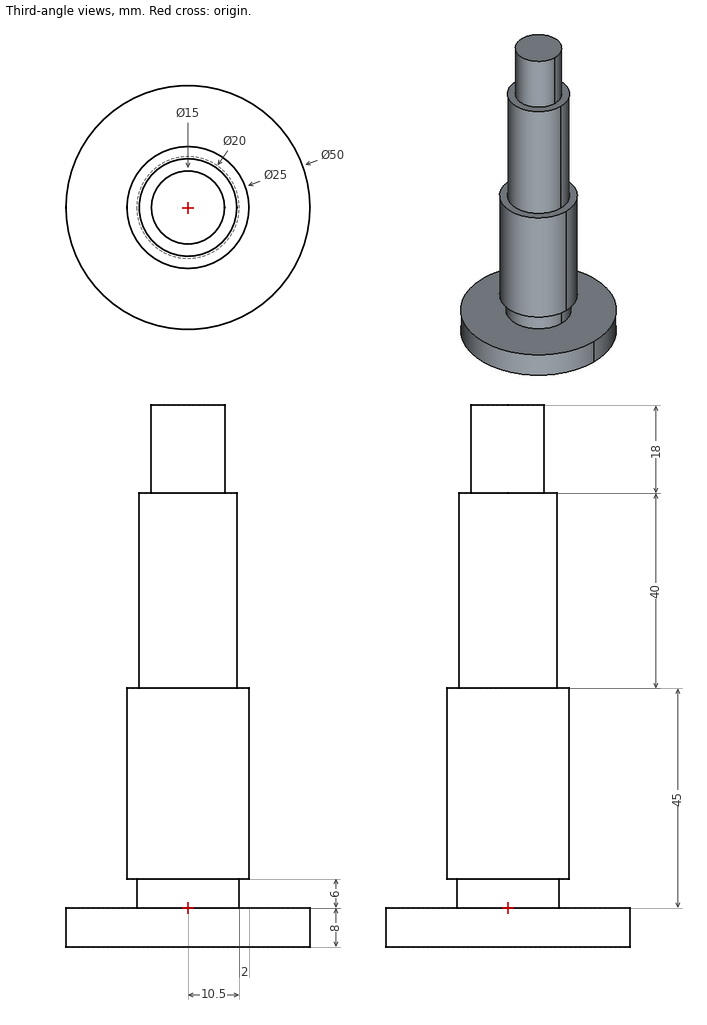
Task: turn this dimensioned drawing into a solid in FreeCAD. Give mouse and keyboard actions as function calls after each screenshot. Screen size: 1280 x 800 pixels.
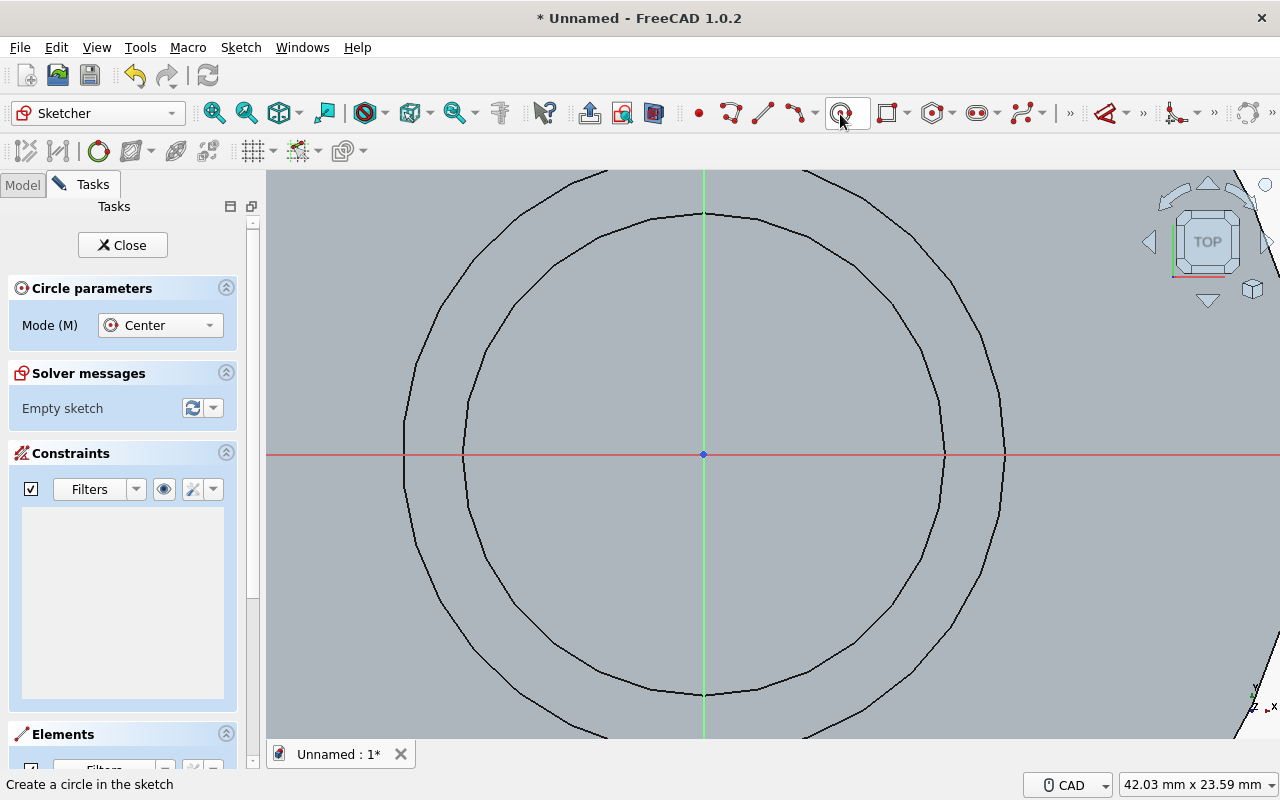
click(704, 454)
move(832, 327)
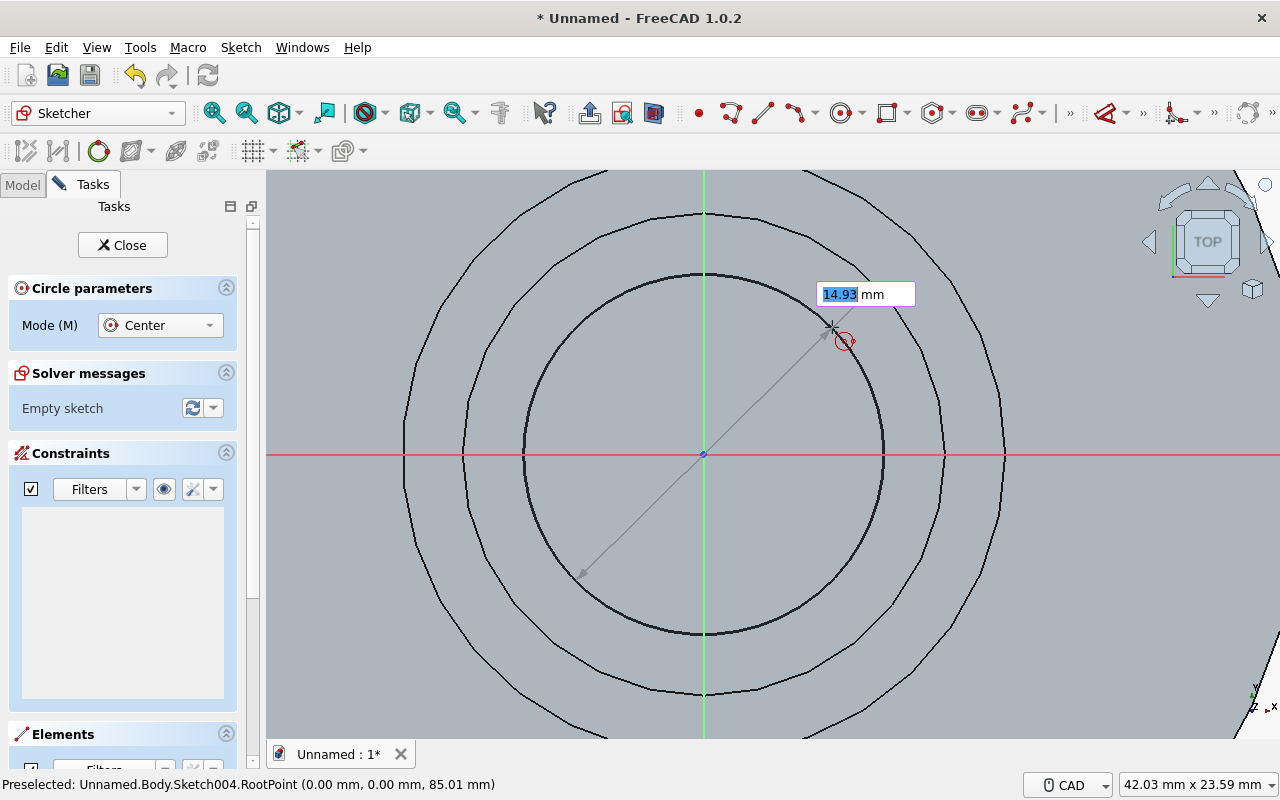
text(15)
key(Return)
key(Escape)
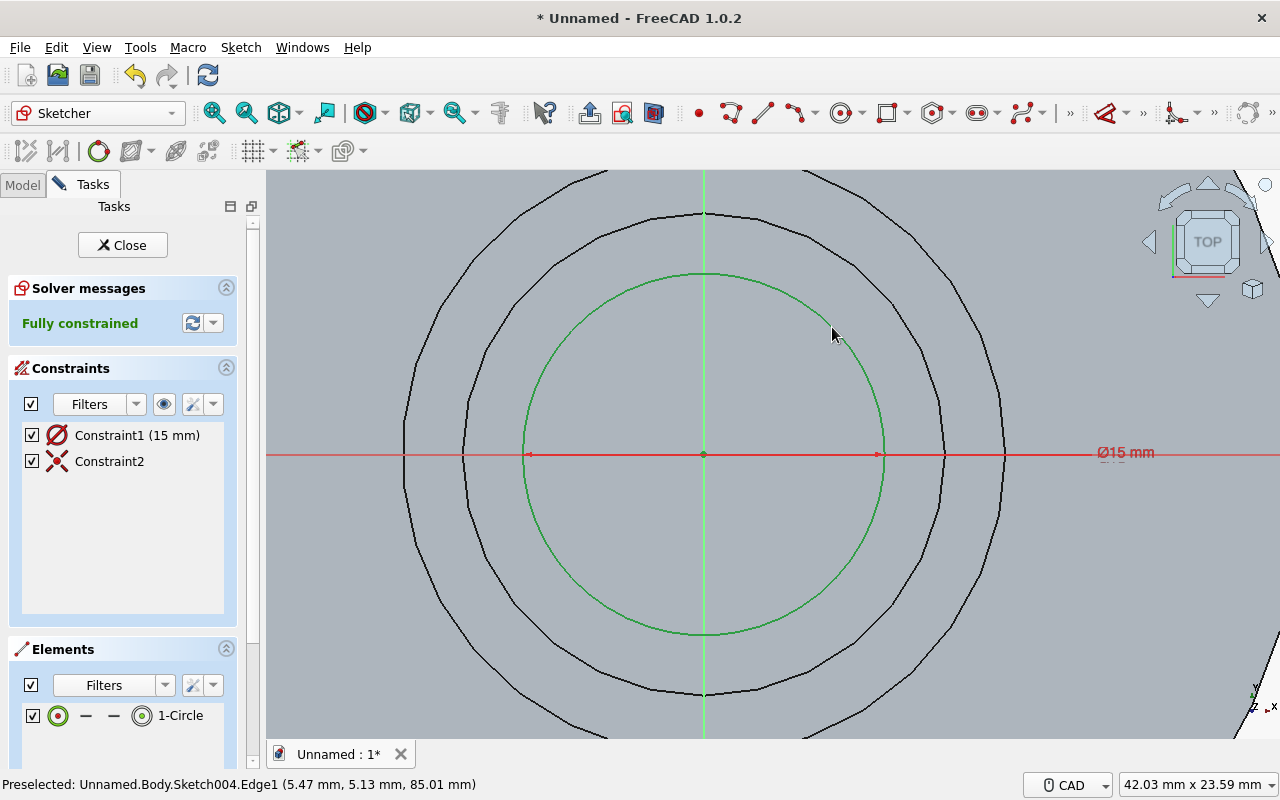
click(123, 245)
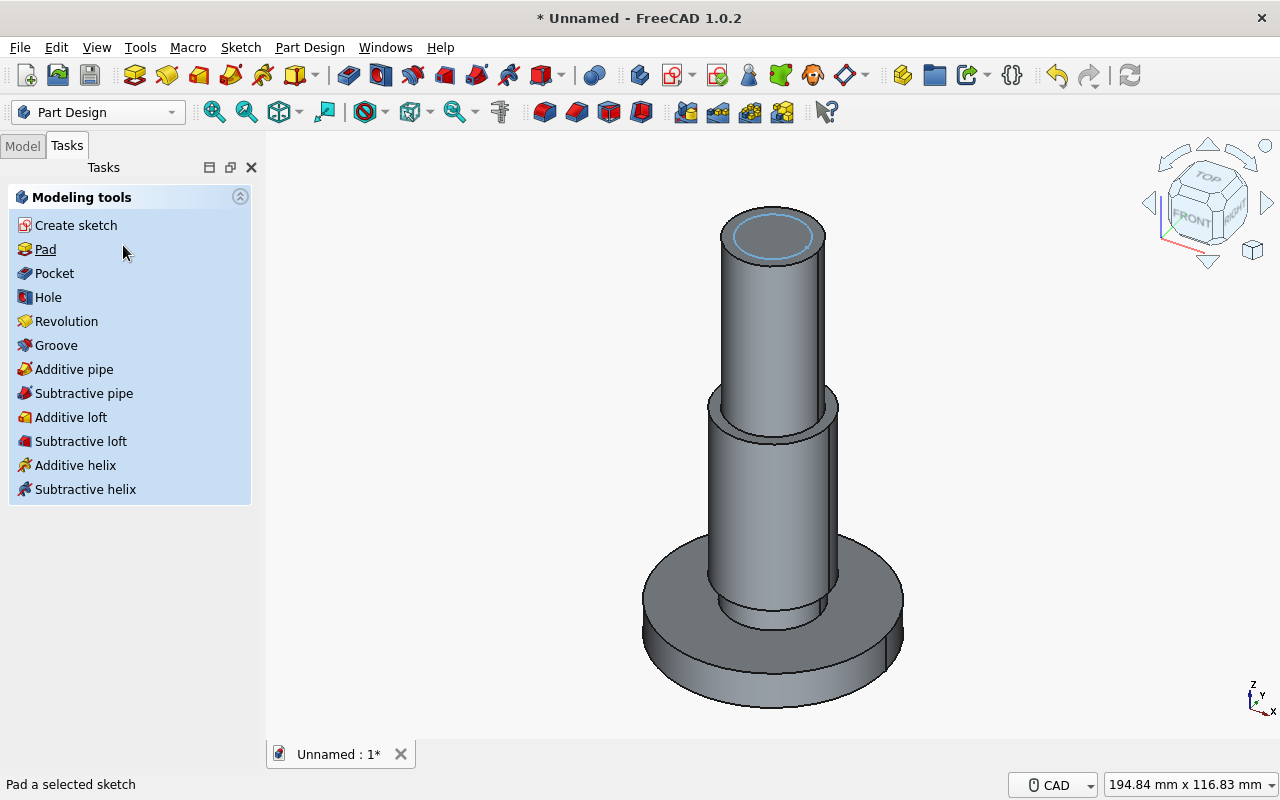
click(136, 76)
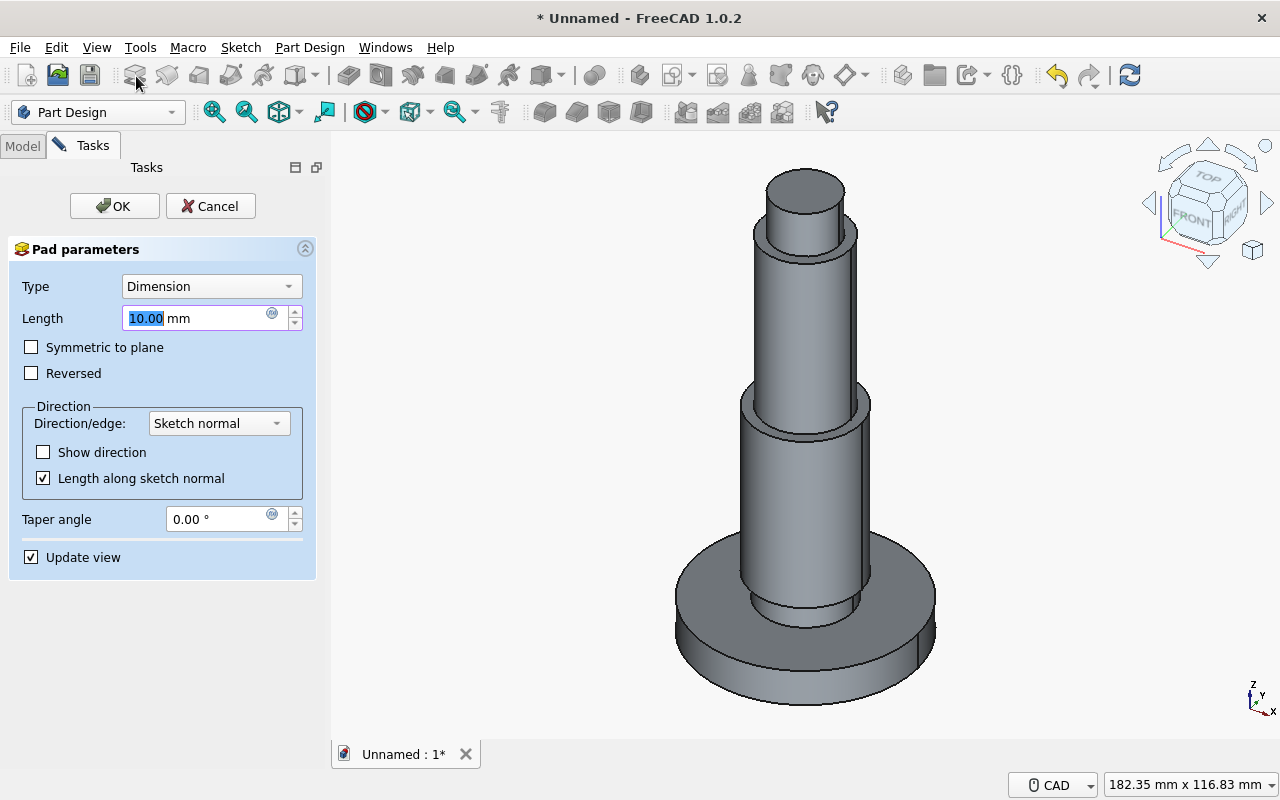
text(18)
key(Tab)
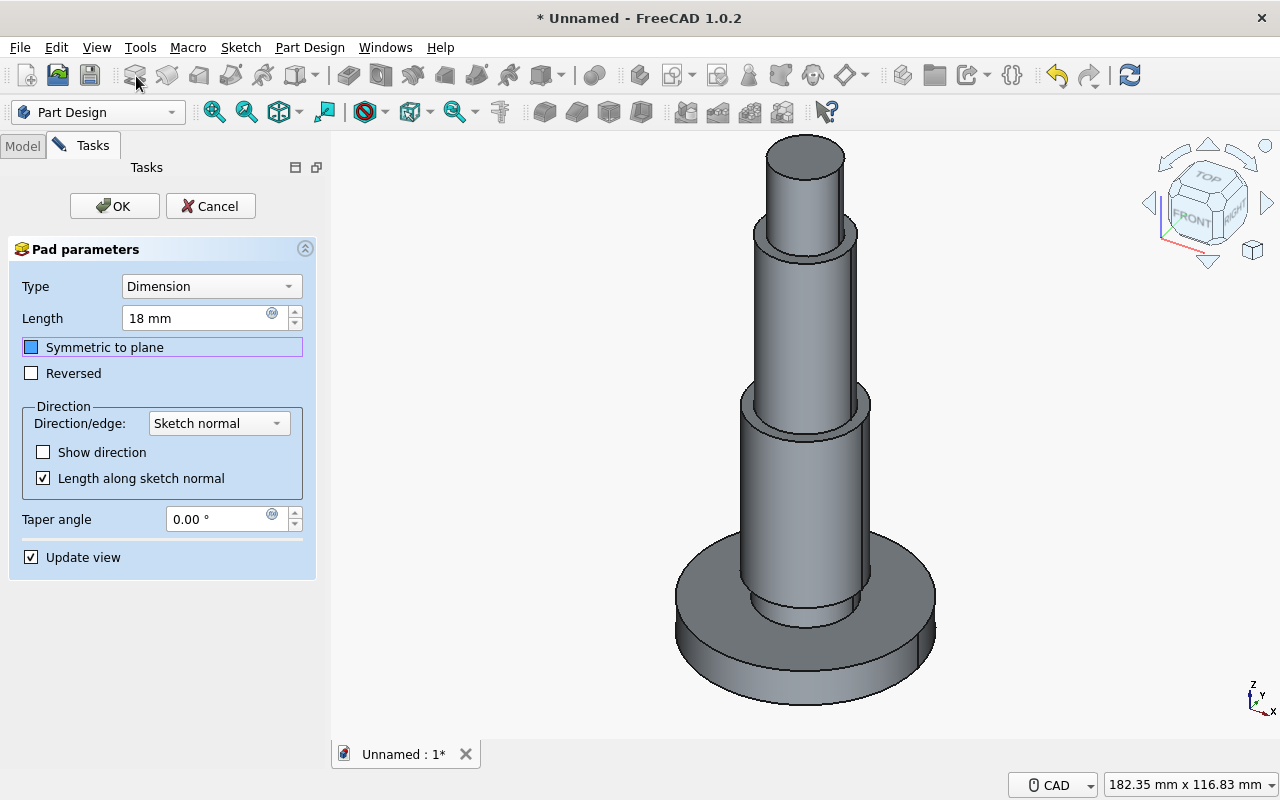
click(115, 206)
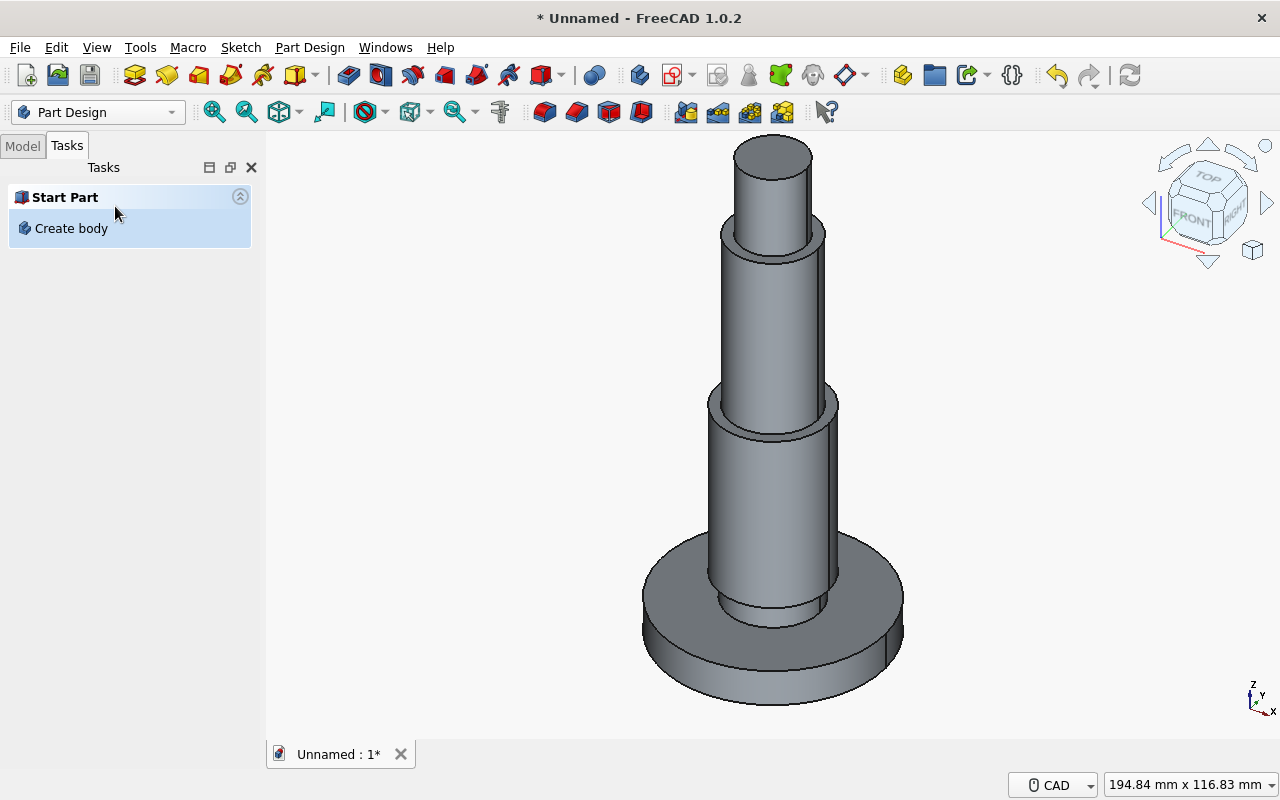
key(0)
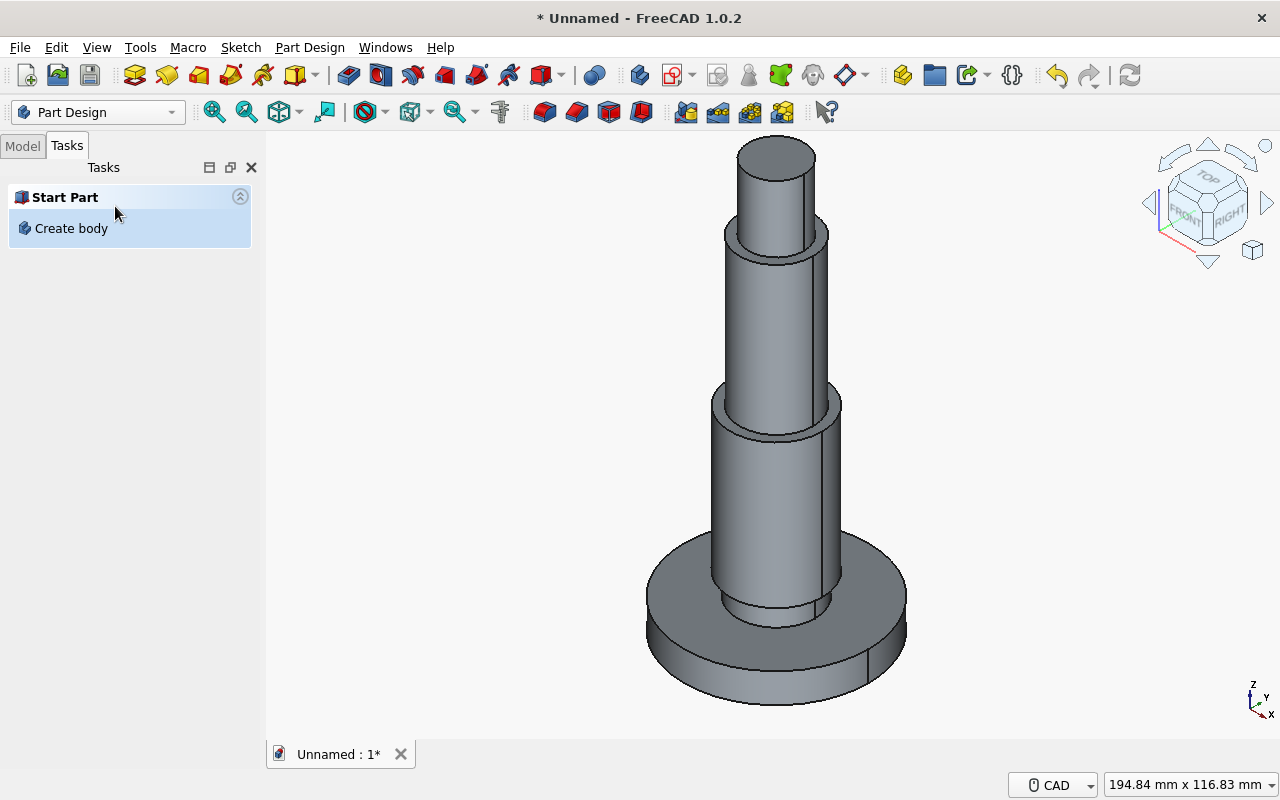
click(216, 112)